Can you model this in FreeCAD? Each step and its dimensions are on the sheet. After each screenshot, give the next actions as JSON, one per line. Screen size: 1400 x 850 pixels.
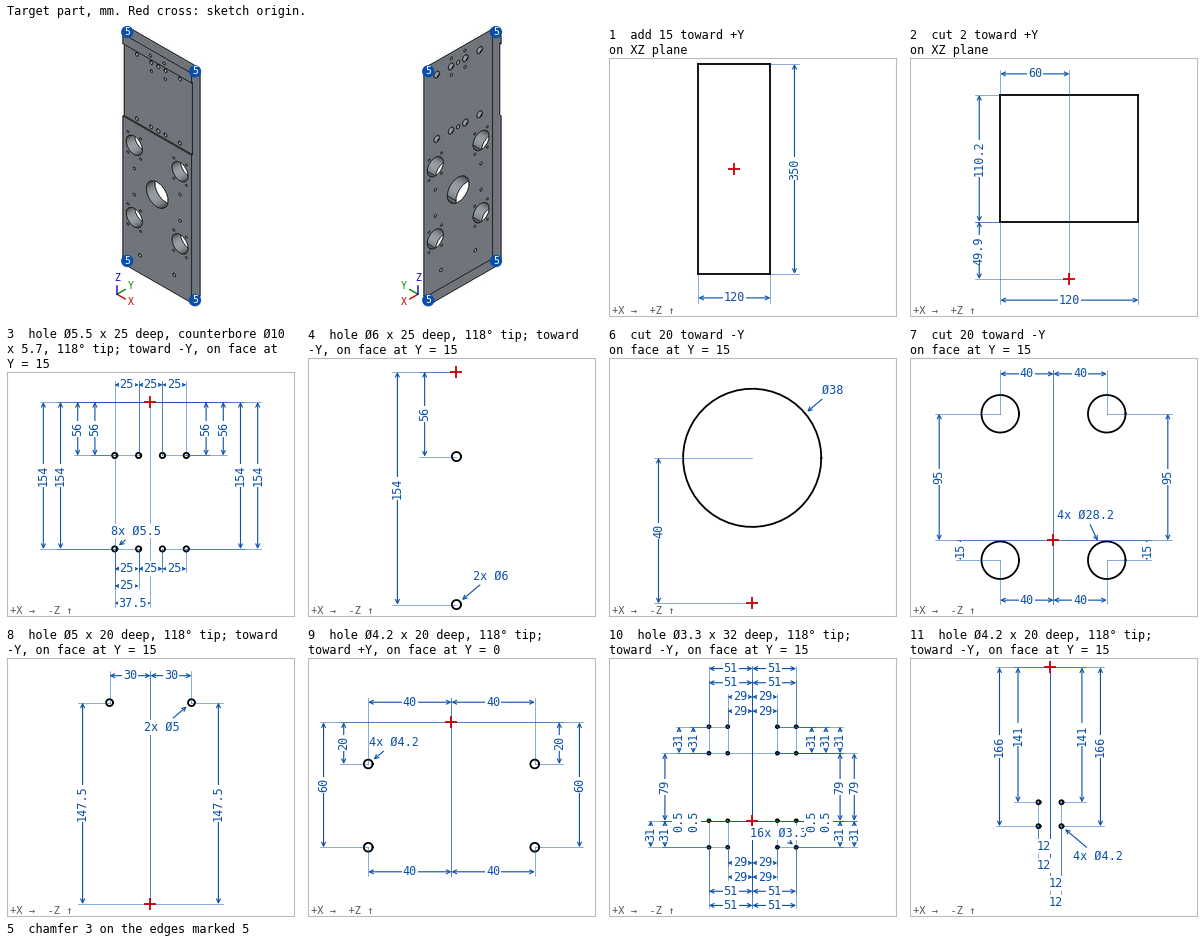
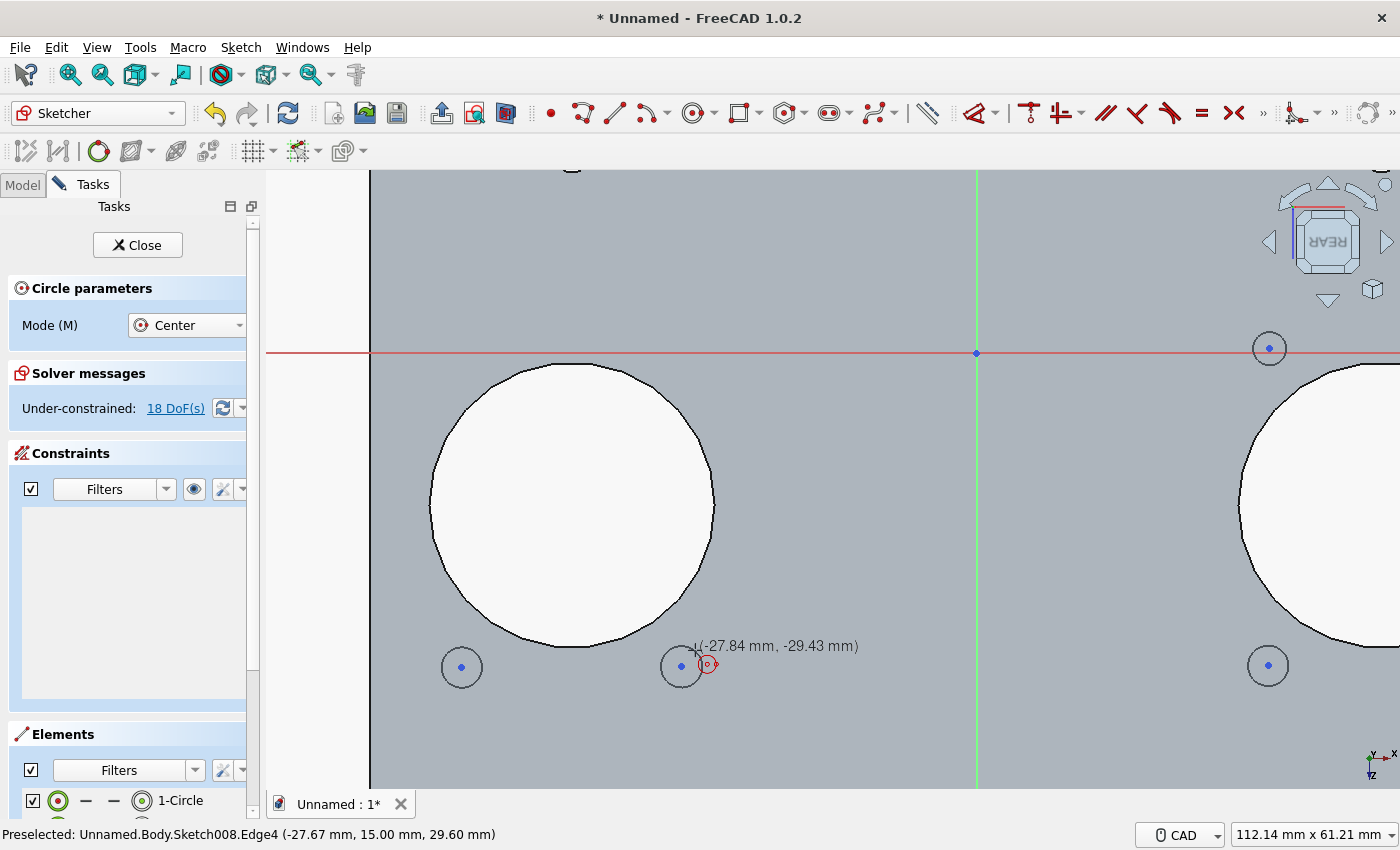
{"action": "scroll", "coordinate": [683, 348], "scroll_direction": "up", "scroll_amount": 6}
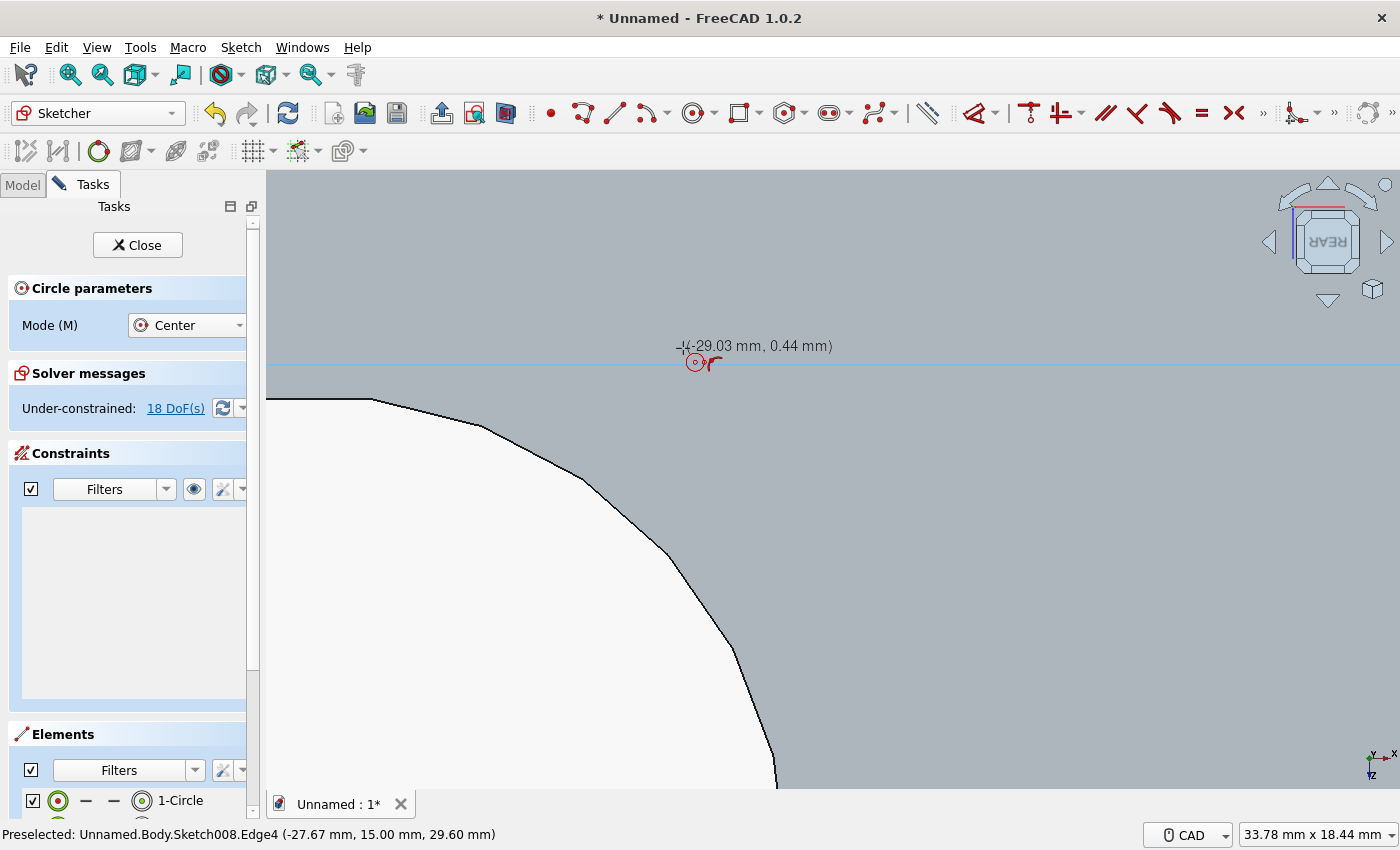
{"action": "left_click", "coordinate": [683, 348]}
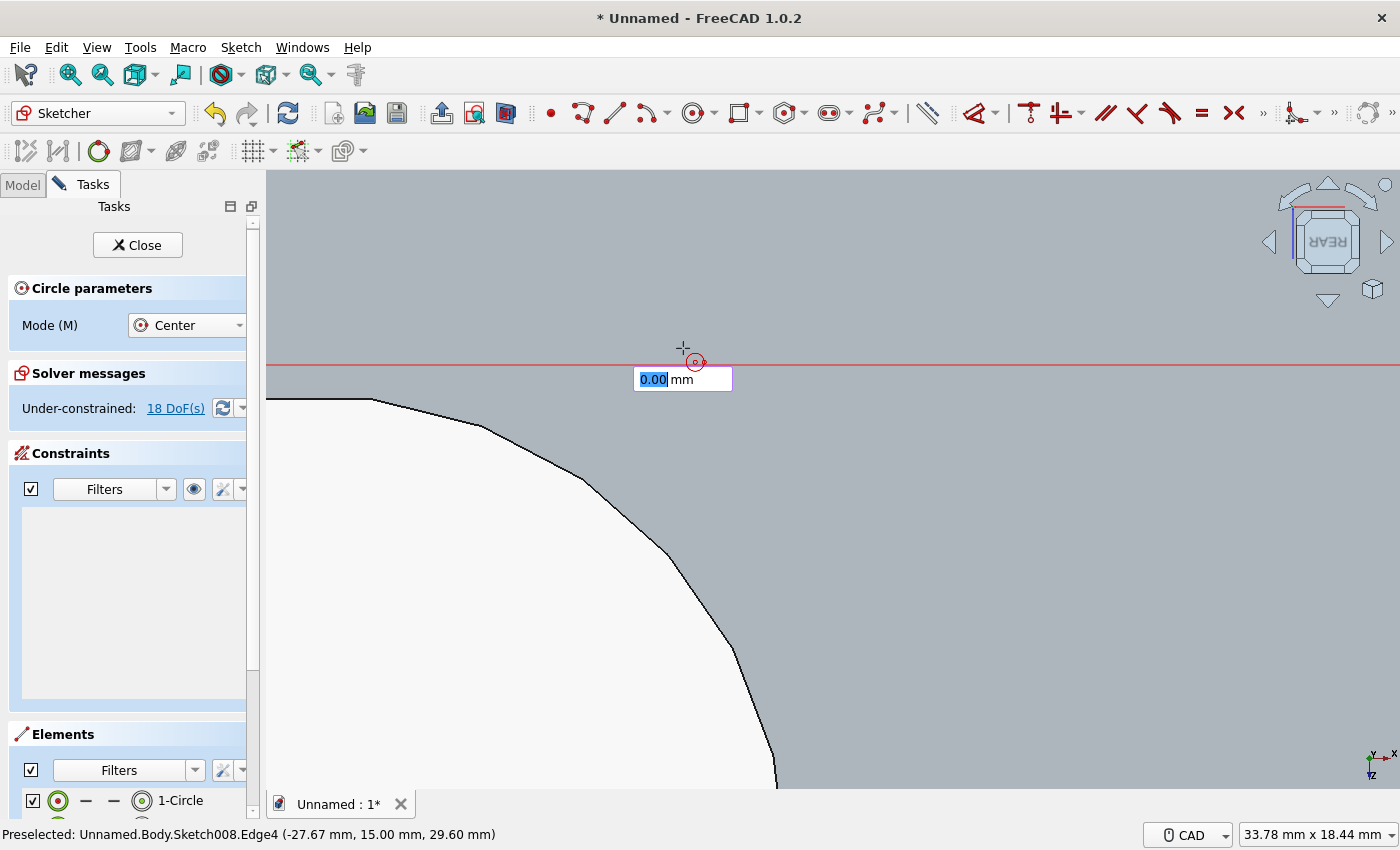
{"action": "scroll", "coordinate": [693, 596], "scroll_direction": "down", "scroll_amount": 13}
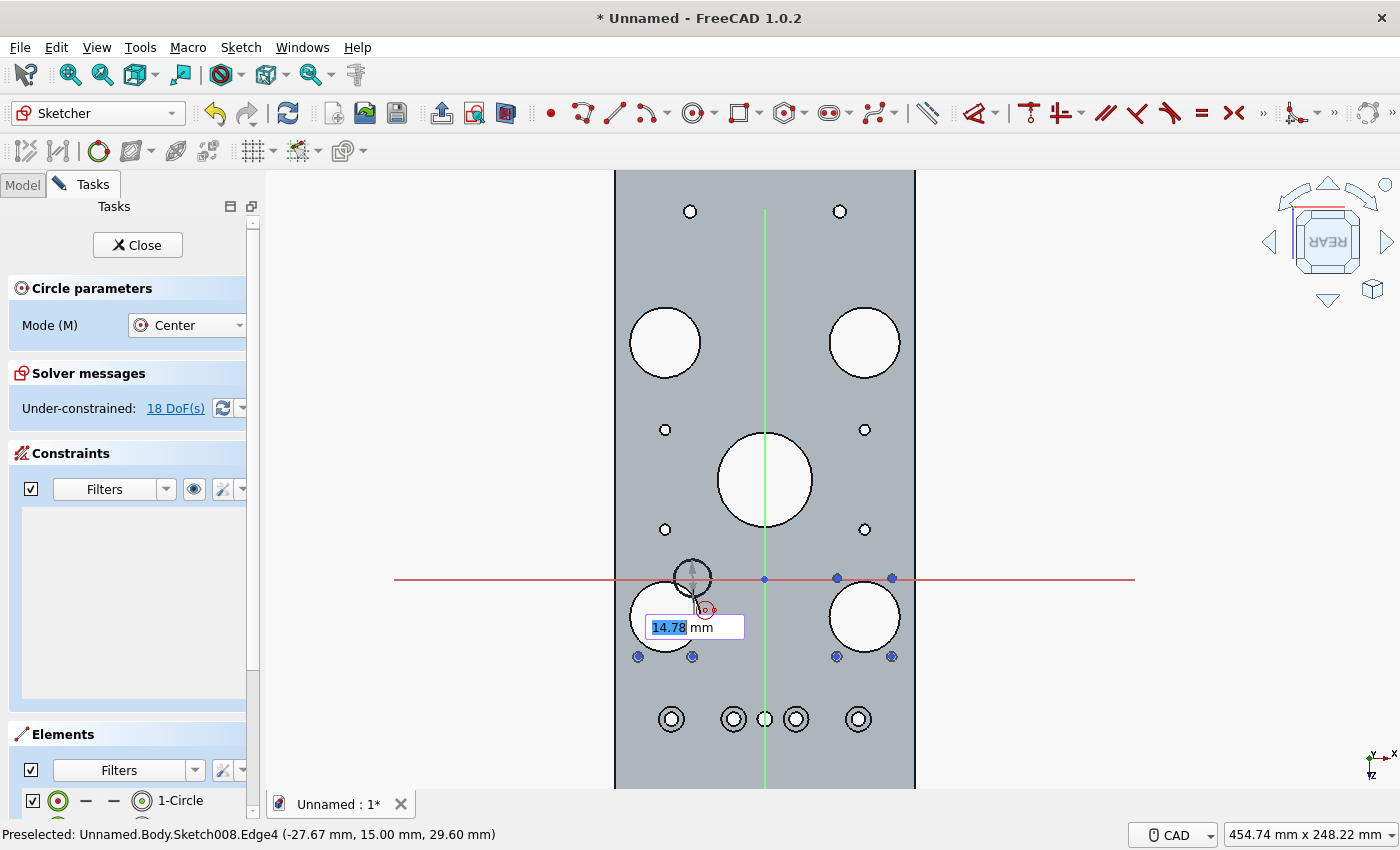
{"action": "scroll", "coordinate": [696, 575], "scroll_direction": "up", "scroll_amount": 7}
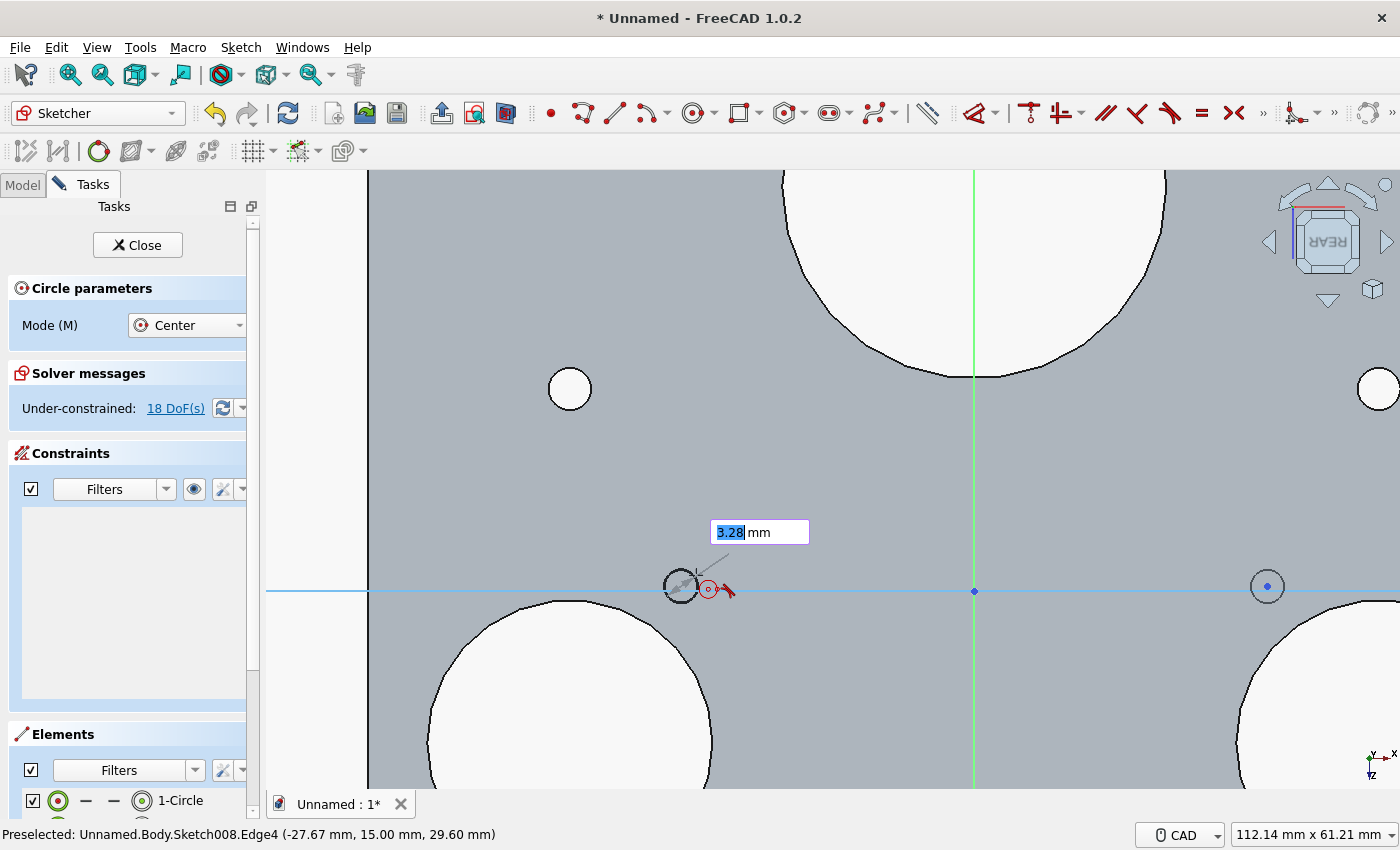
{"action": "left_click", "coordinate": [693, 574]}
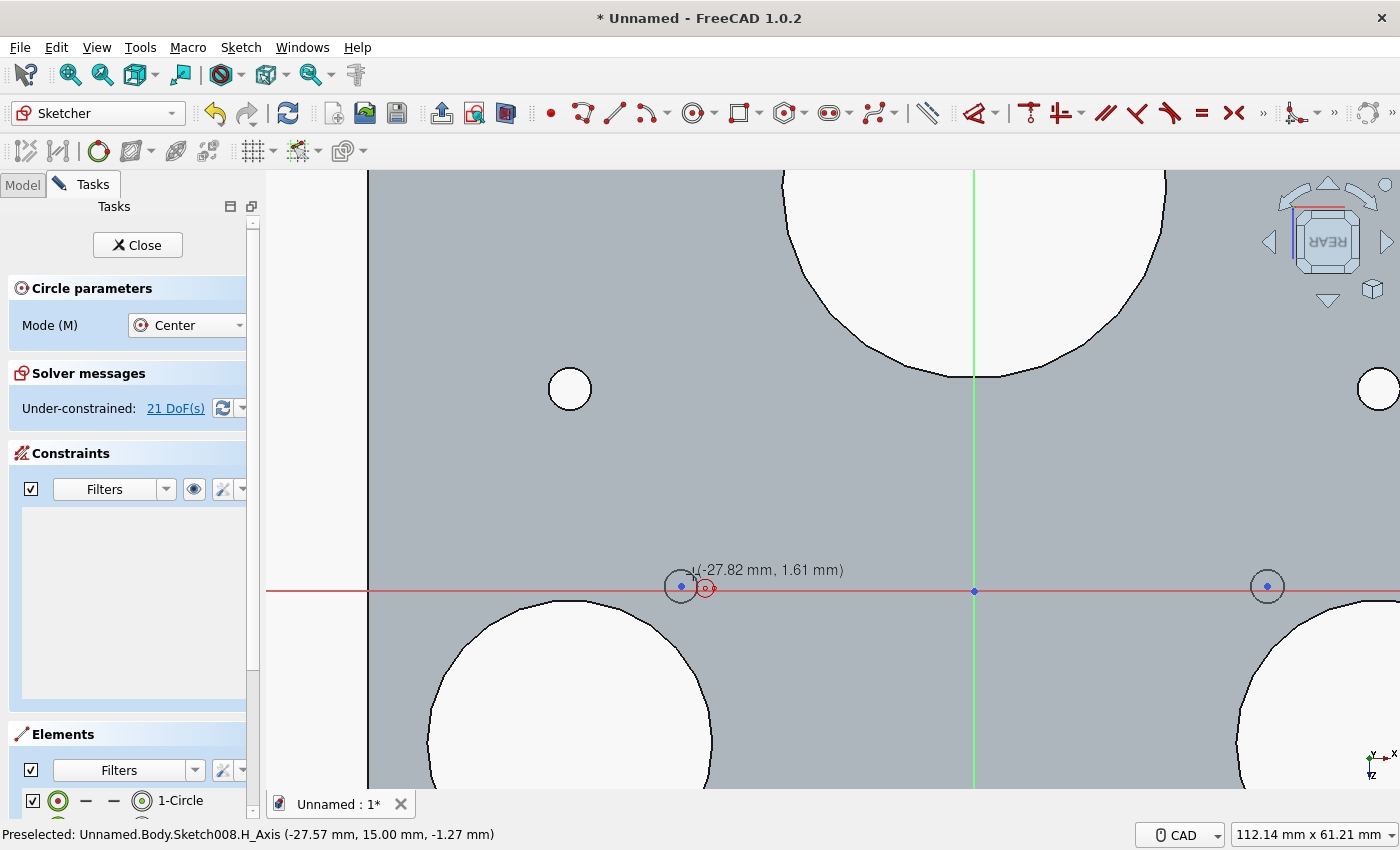
{"action": "scroll", "coordinate": [459, 586], "scroll_direction": "up", "scroll_amount": 6}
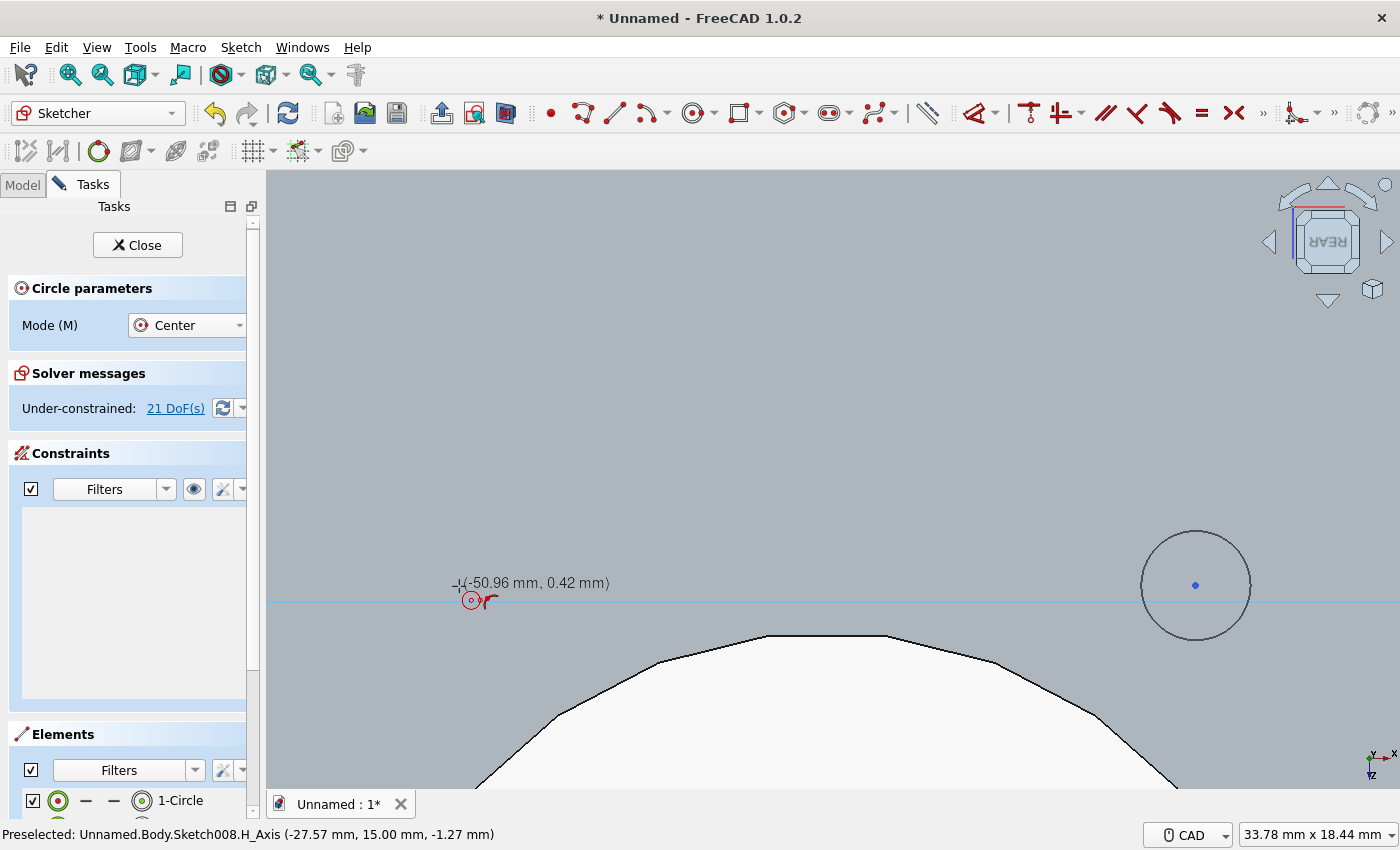
{"action": "left_click", "coordinate": [457, 585]}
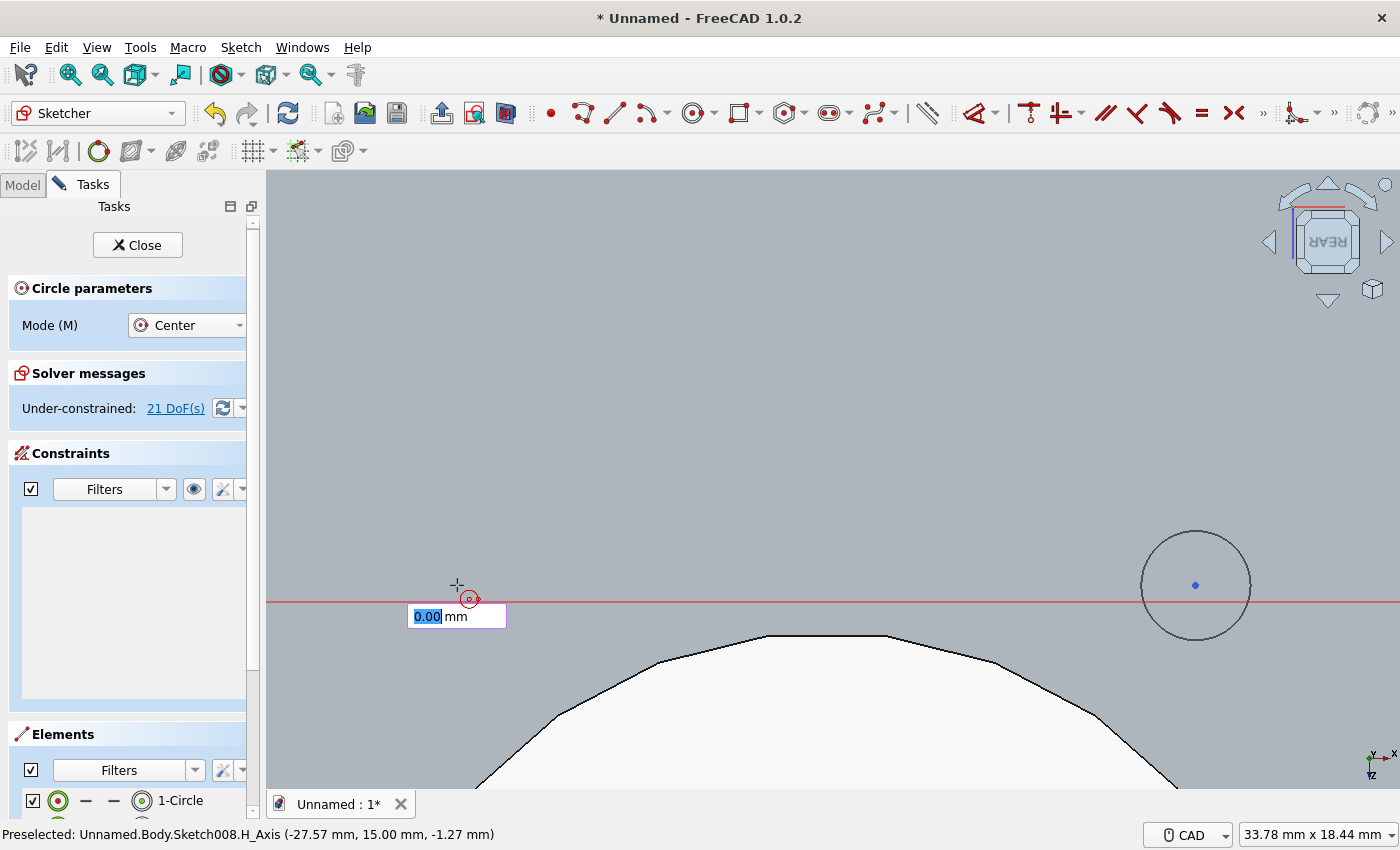
{"action": "scroll", "coordinate": [652, 577], "scroll_direction": "down", "scroll_amount": 13}